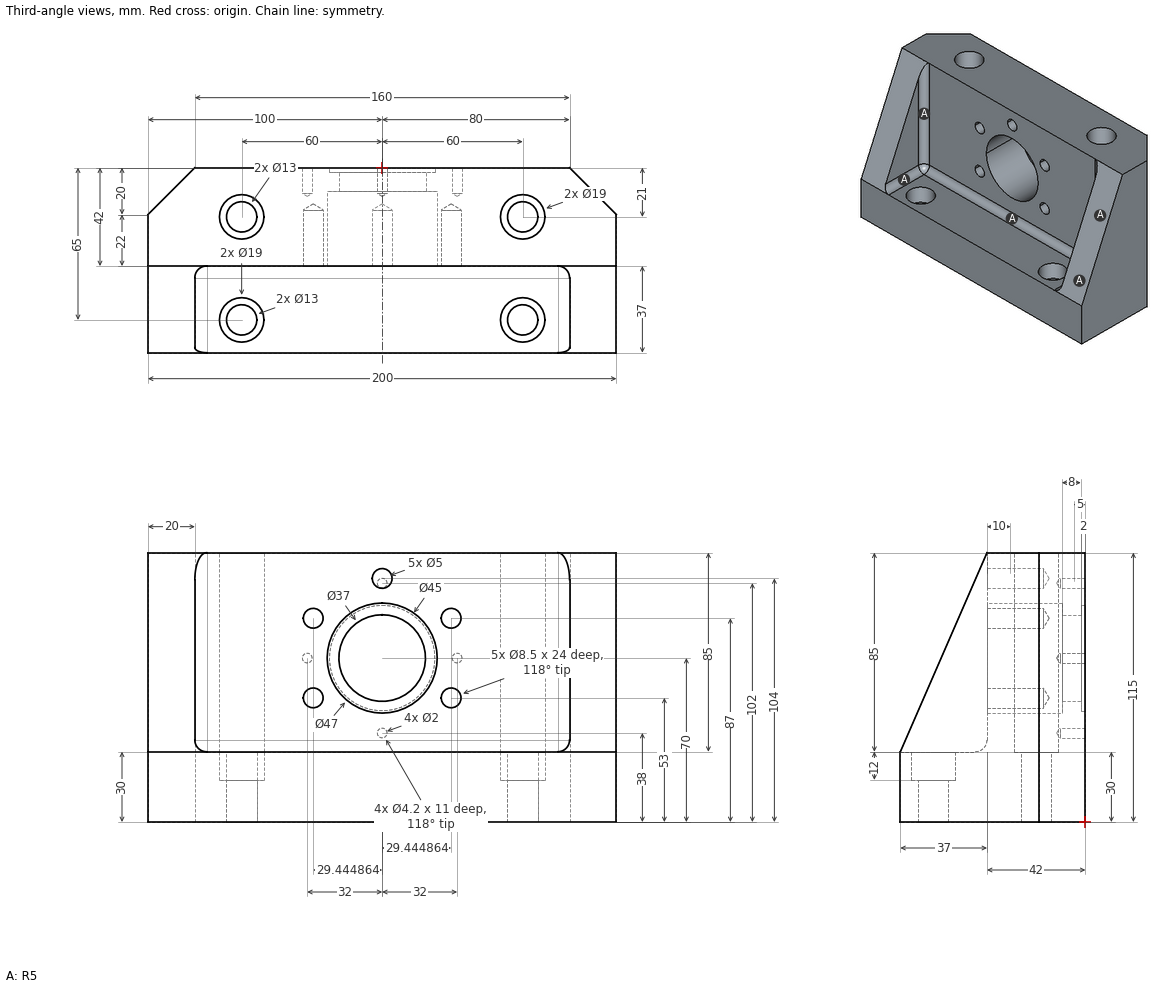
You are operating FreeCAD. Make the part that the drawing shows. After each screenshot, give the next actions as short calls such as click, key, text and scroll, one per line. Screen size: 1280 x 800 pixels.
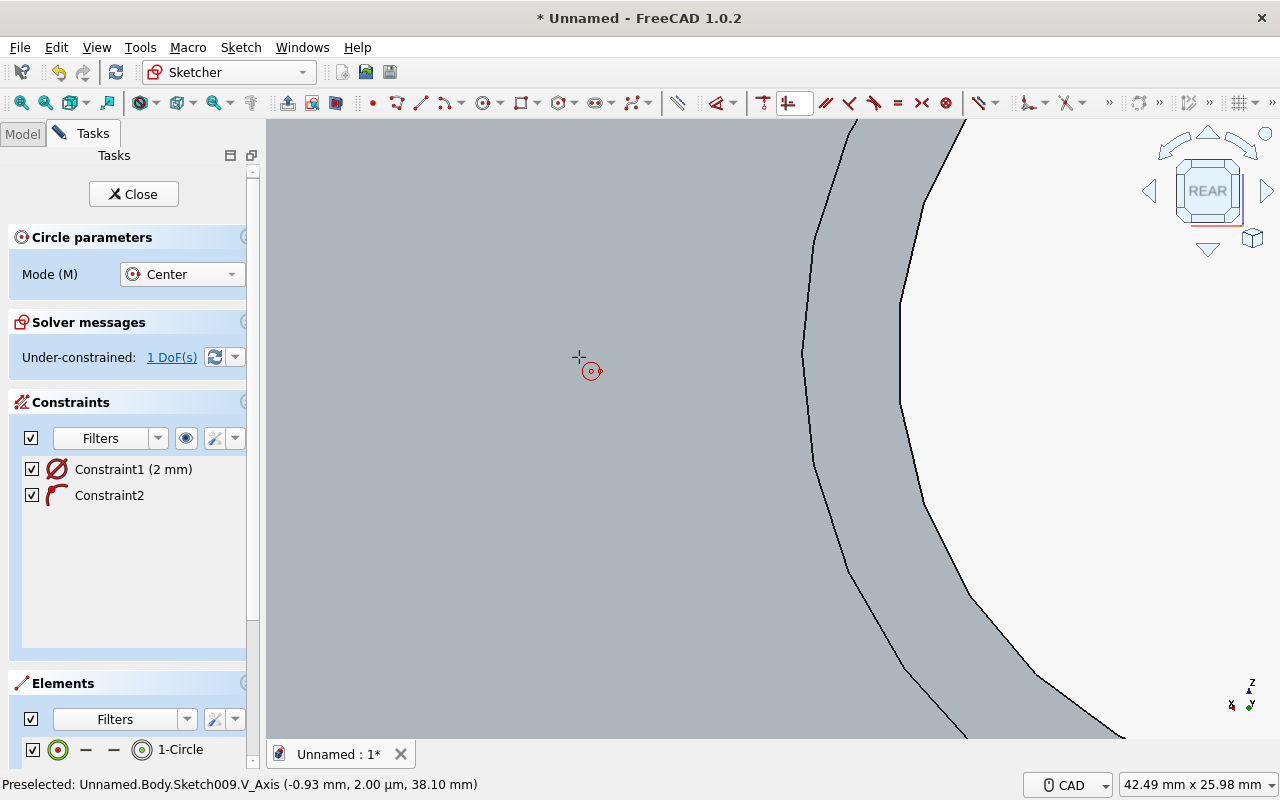
scroll(579, 357, down, 9)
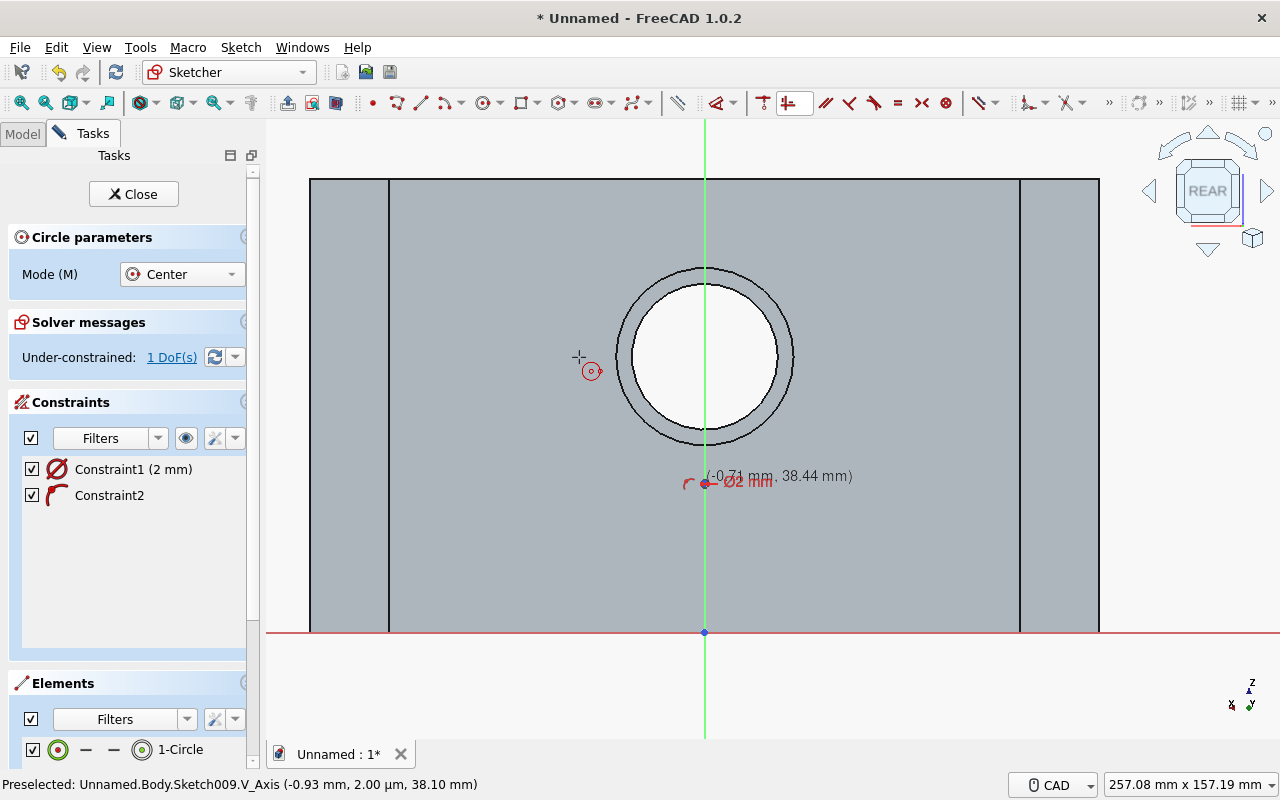
click(579, 357)
move(581, 354)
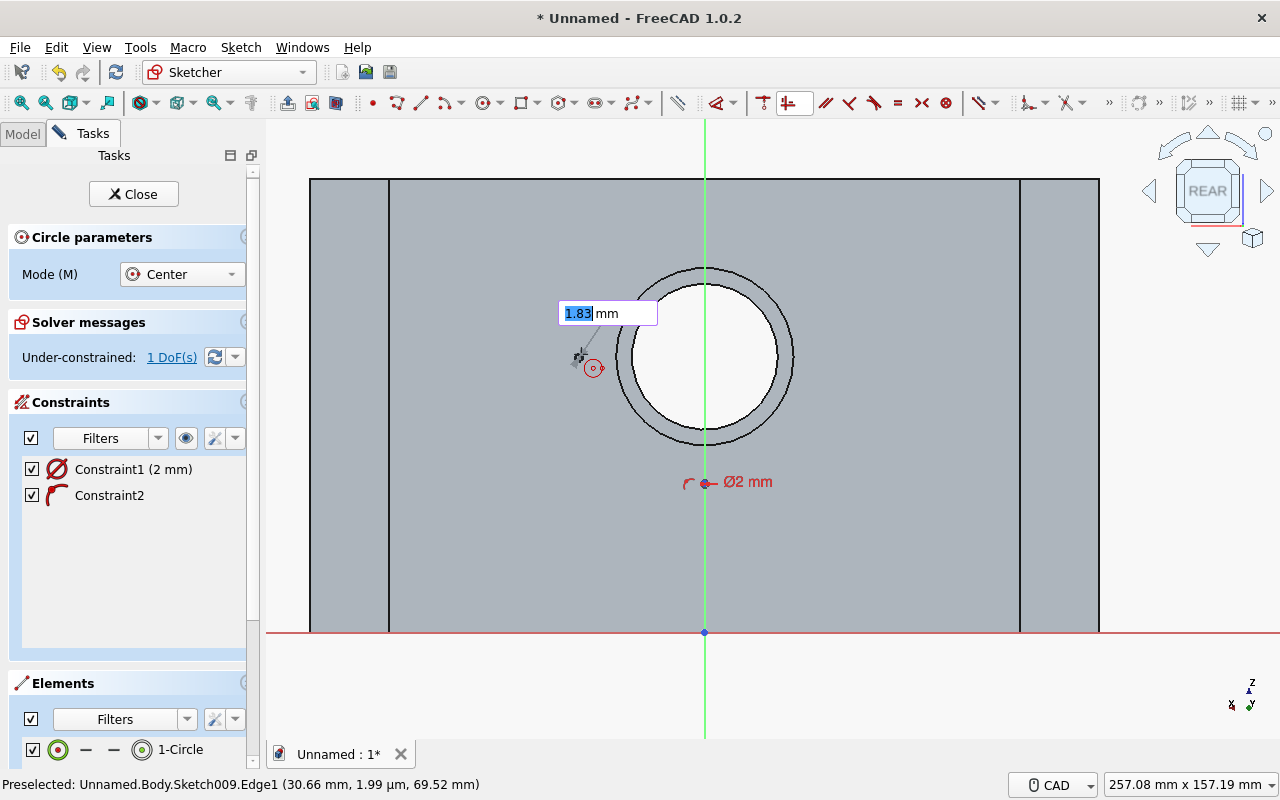
text(2)
key(Return)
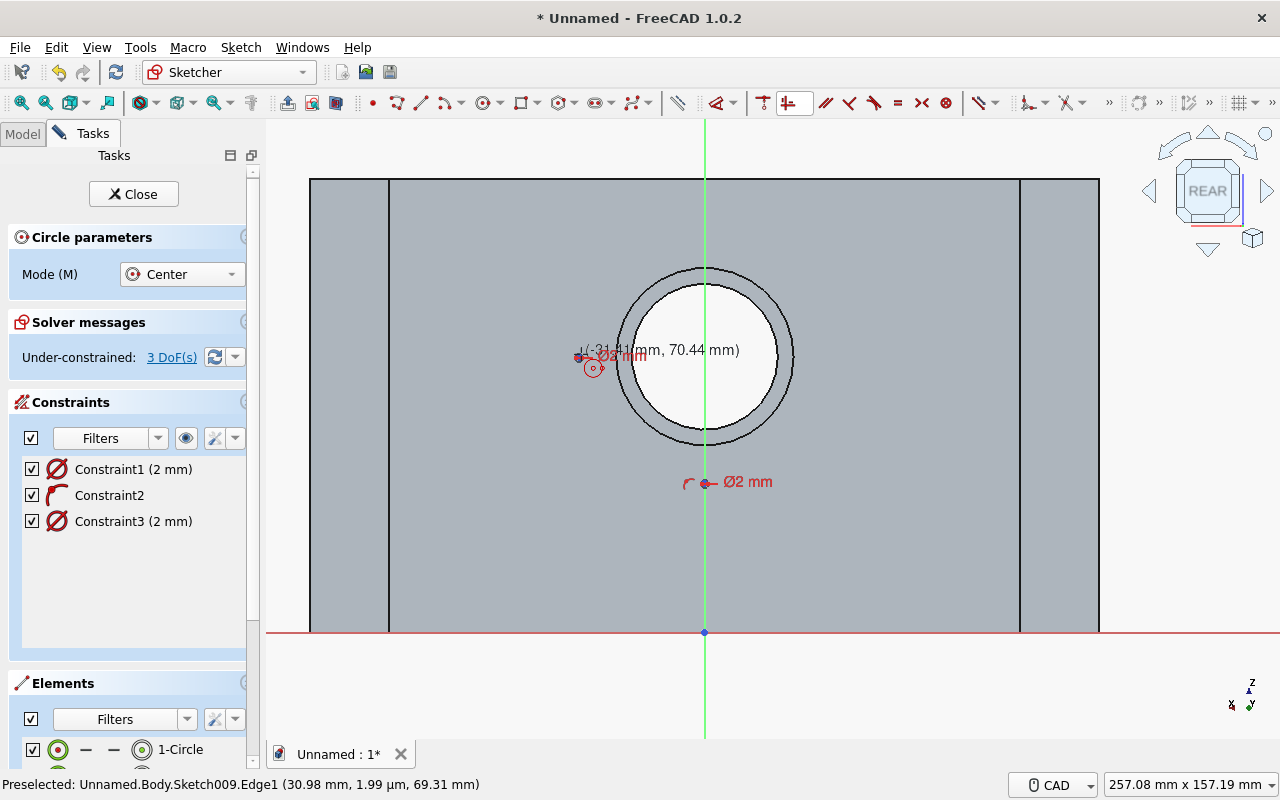
scroll(705, 231, up, 9)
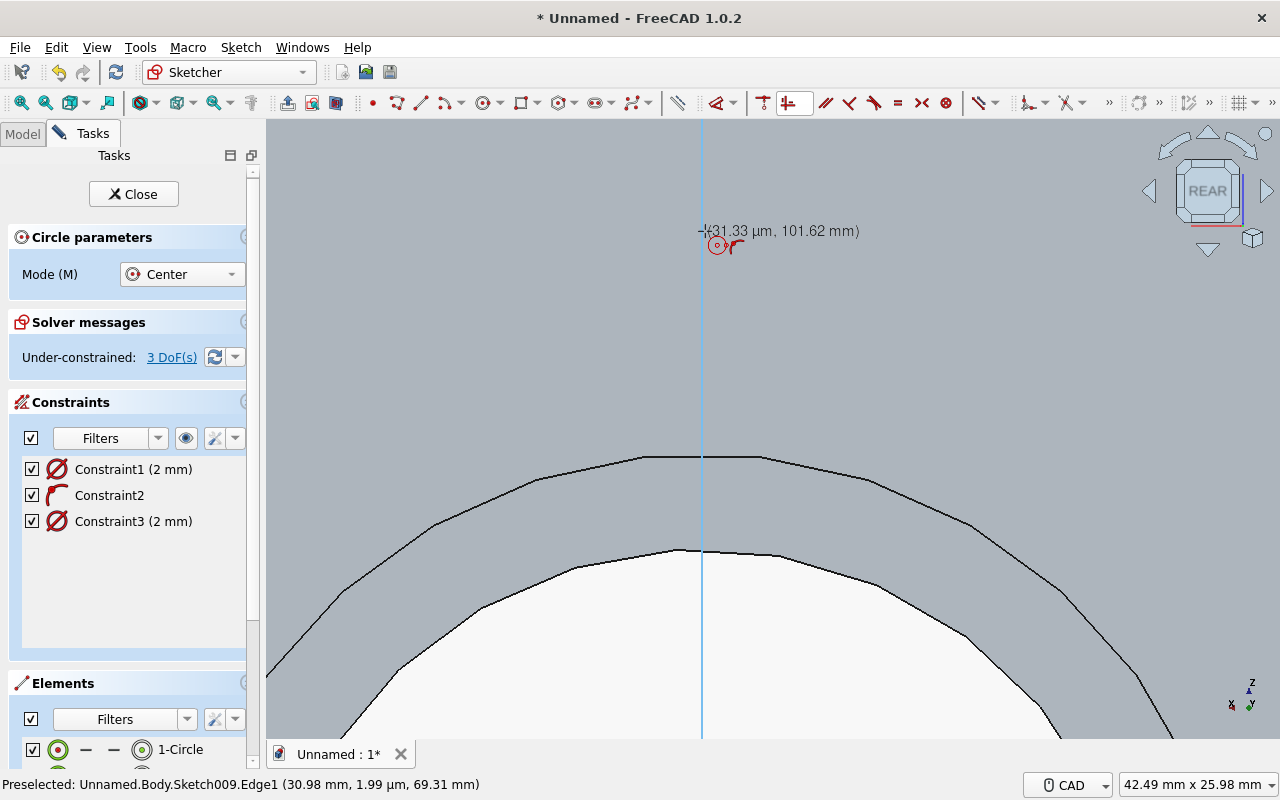
scroll(705, 230, down, 9)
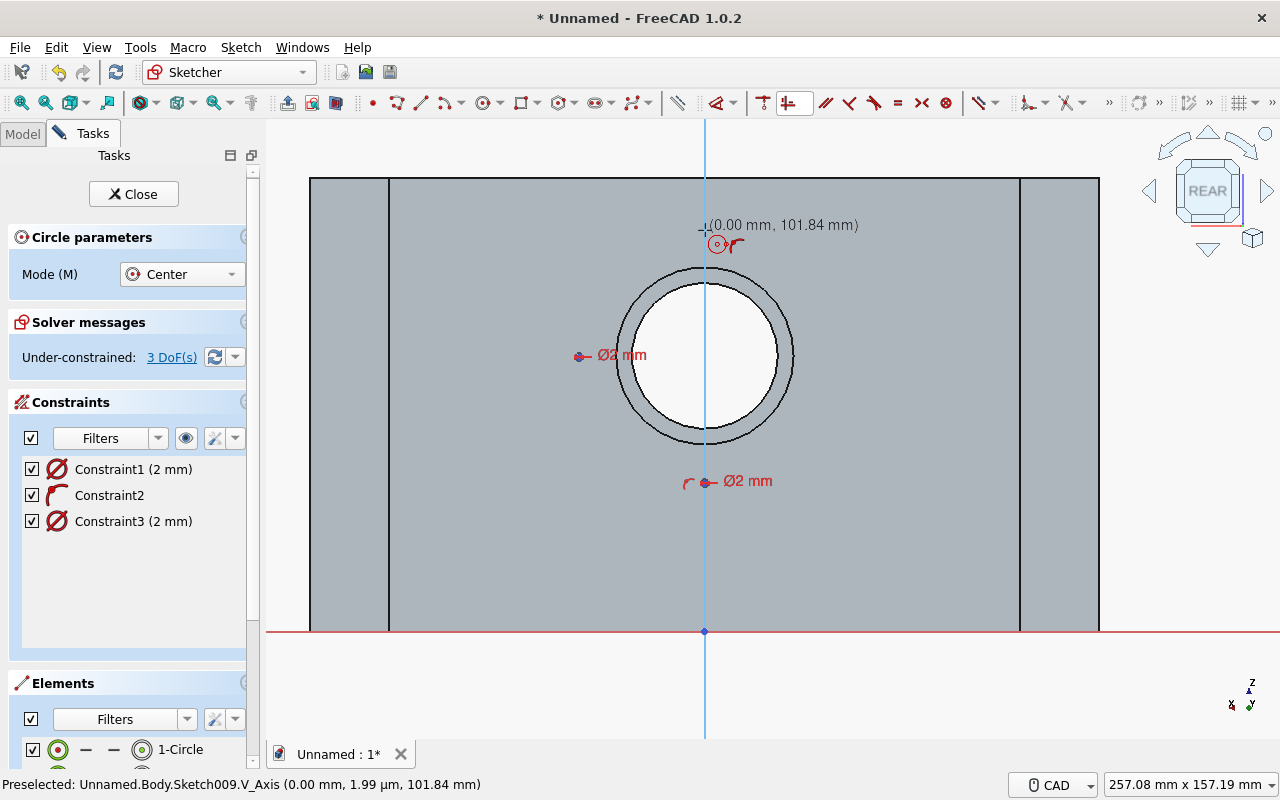
click(705, 230)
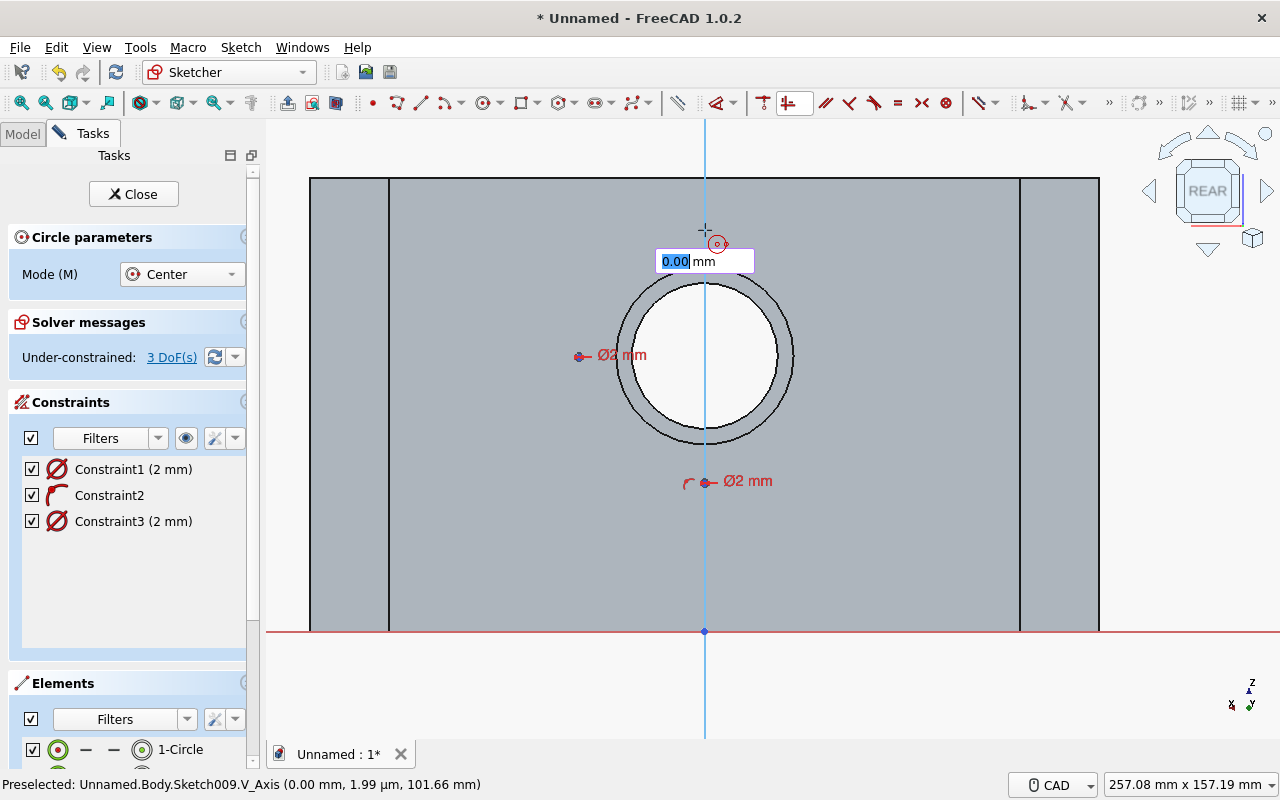
scroll(709, 228, up, 8)
move(705, 229)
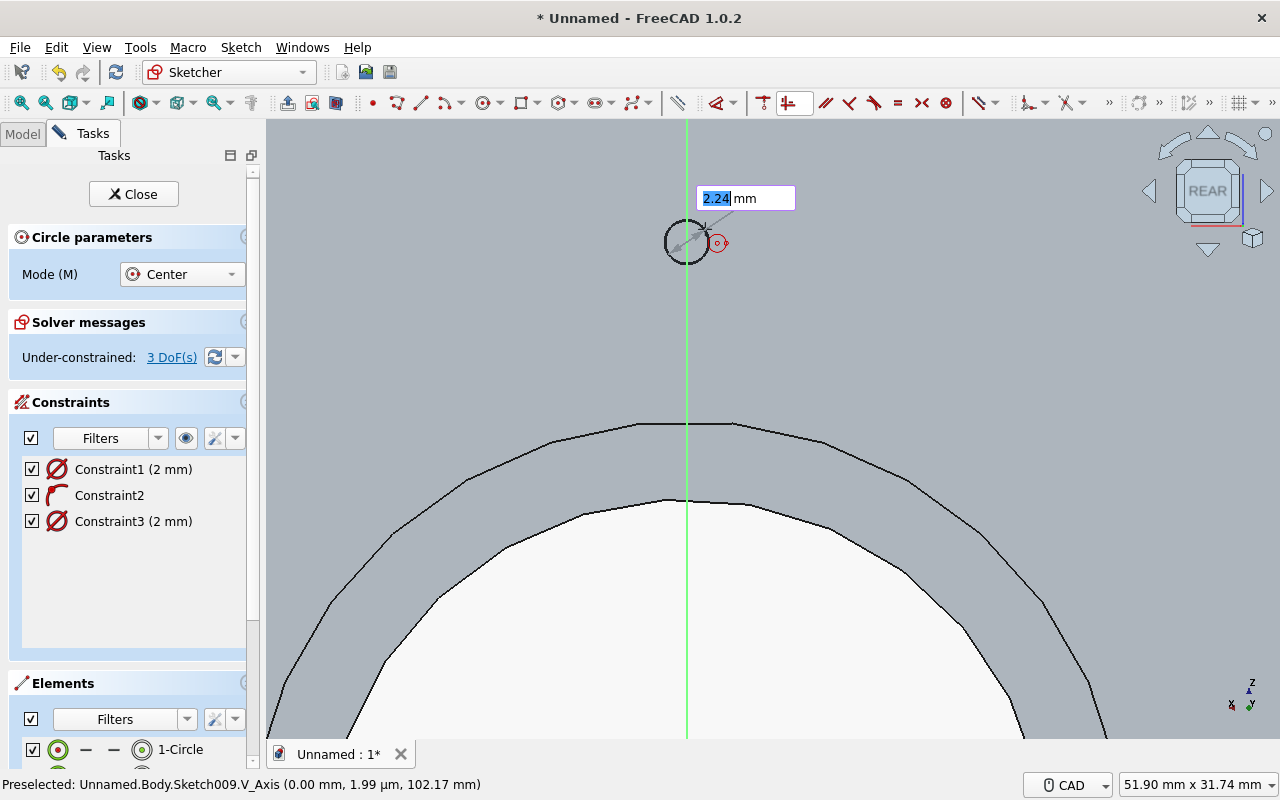
text(2)
key(Return)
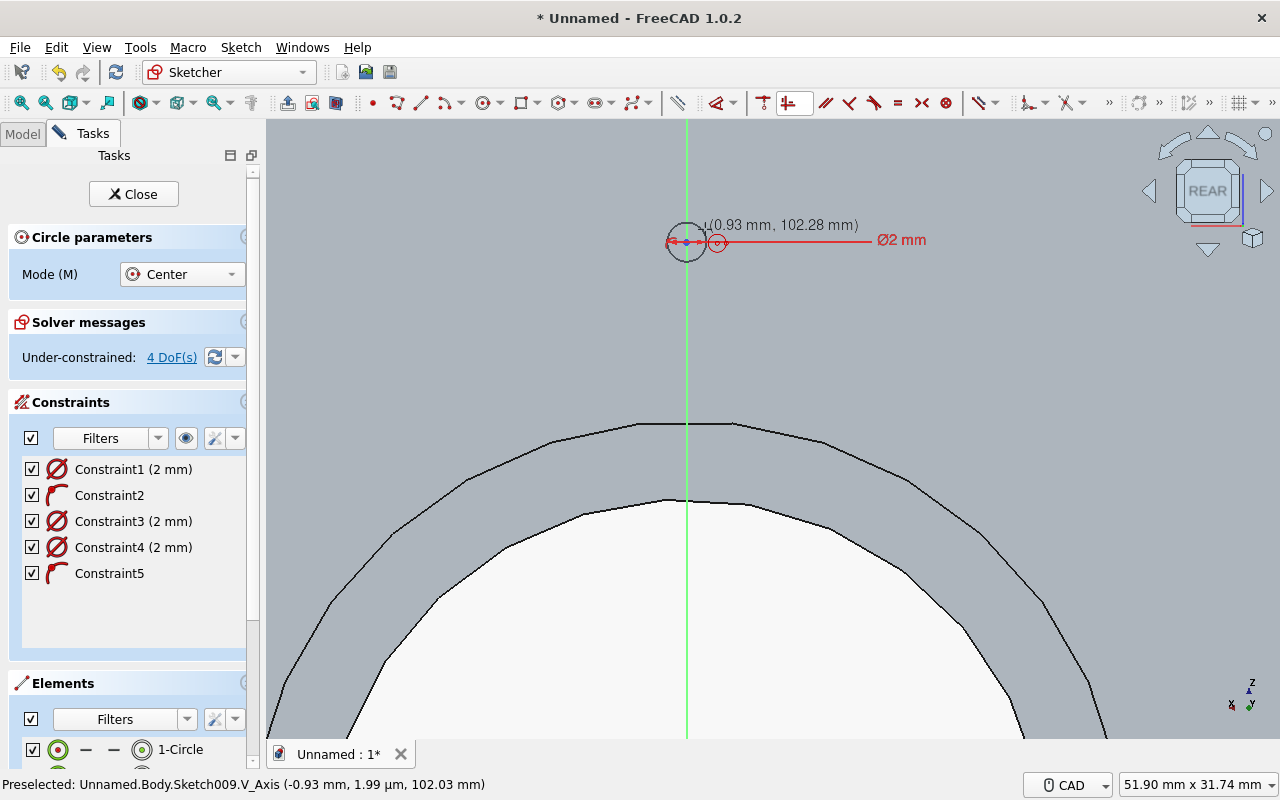
scroll(709, 228, down, 8)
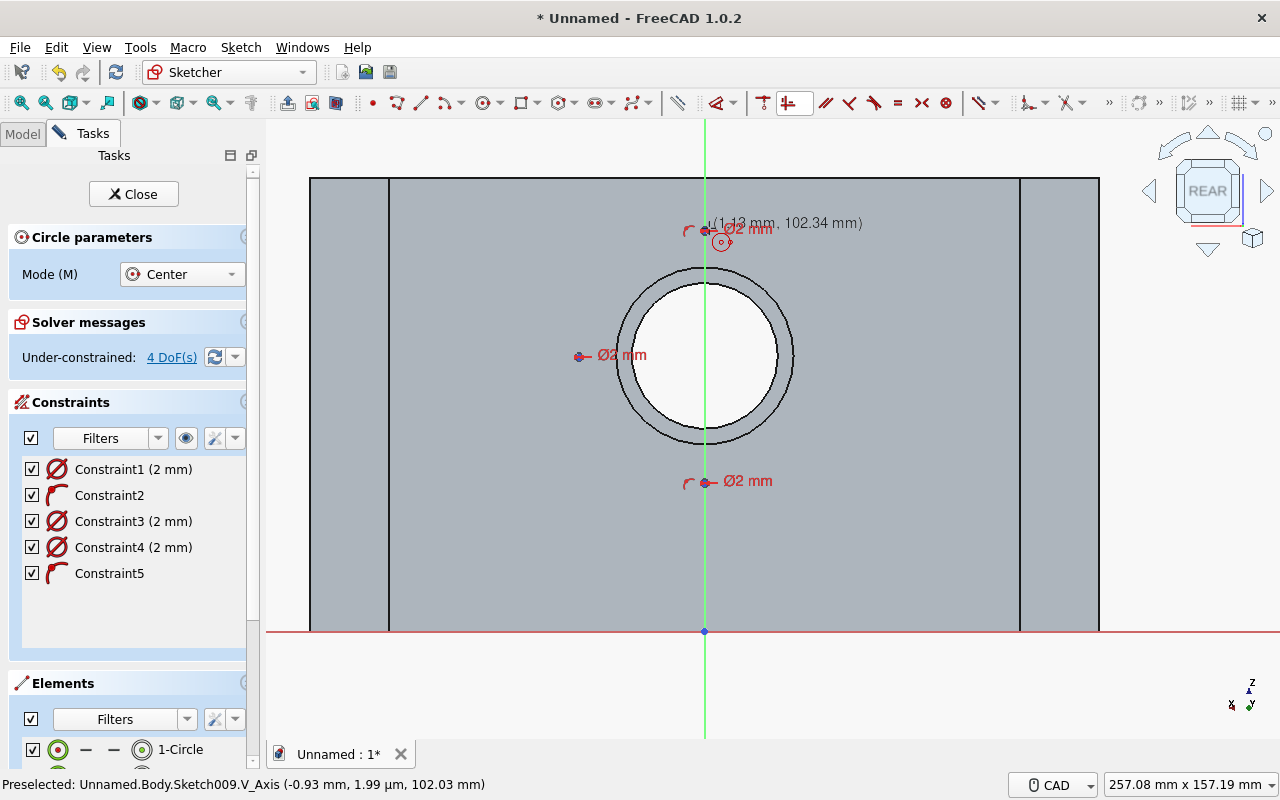
scroll(831, 356, up, 9)